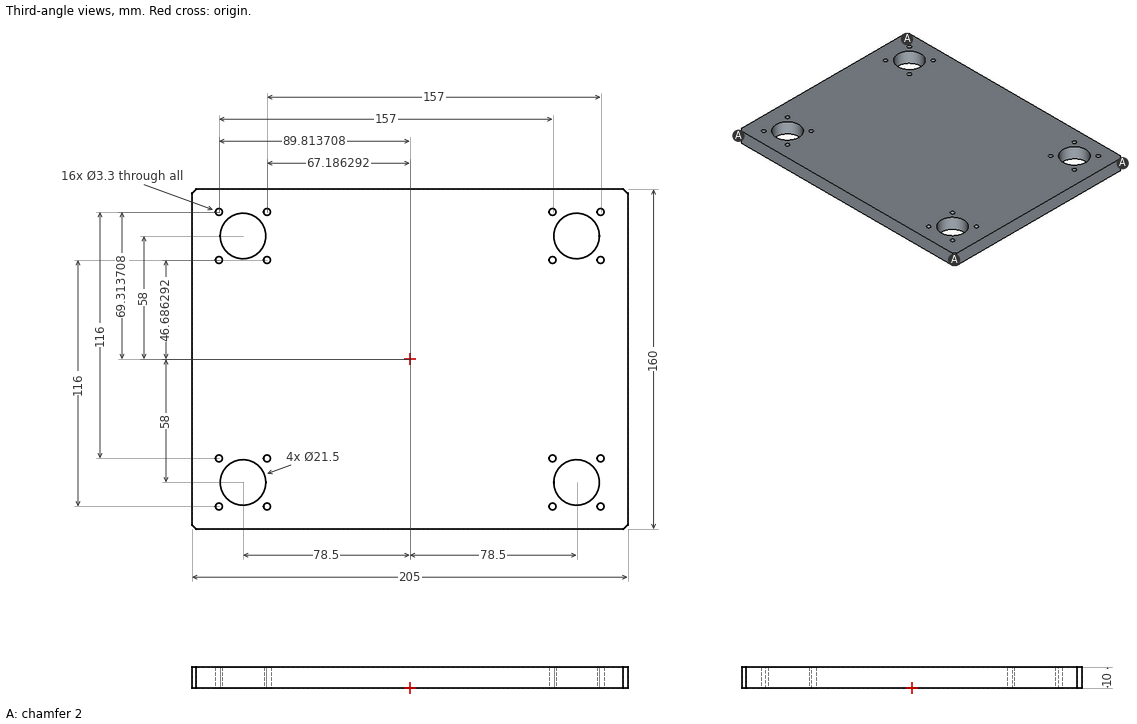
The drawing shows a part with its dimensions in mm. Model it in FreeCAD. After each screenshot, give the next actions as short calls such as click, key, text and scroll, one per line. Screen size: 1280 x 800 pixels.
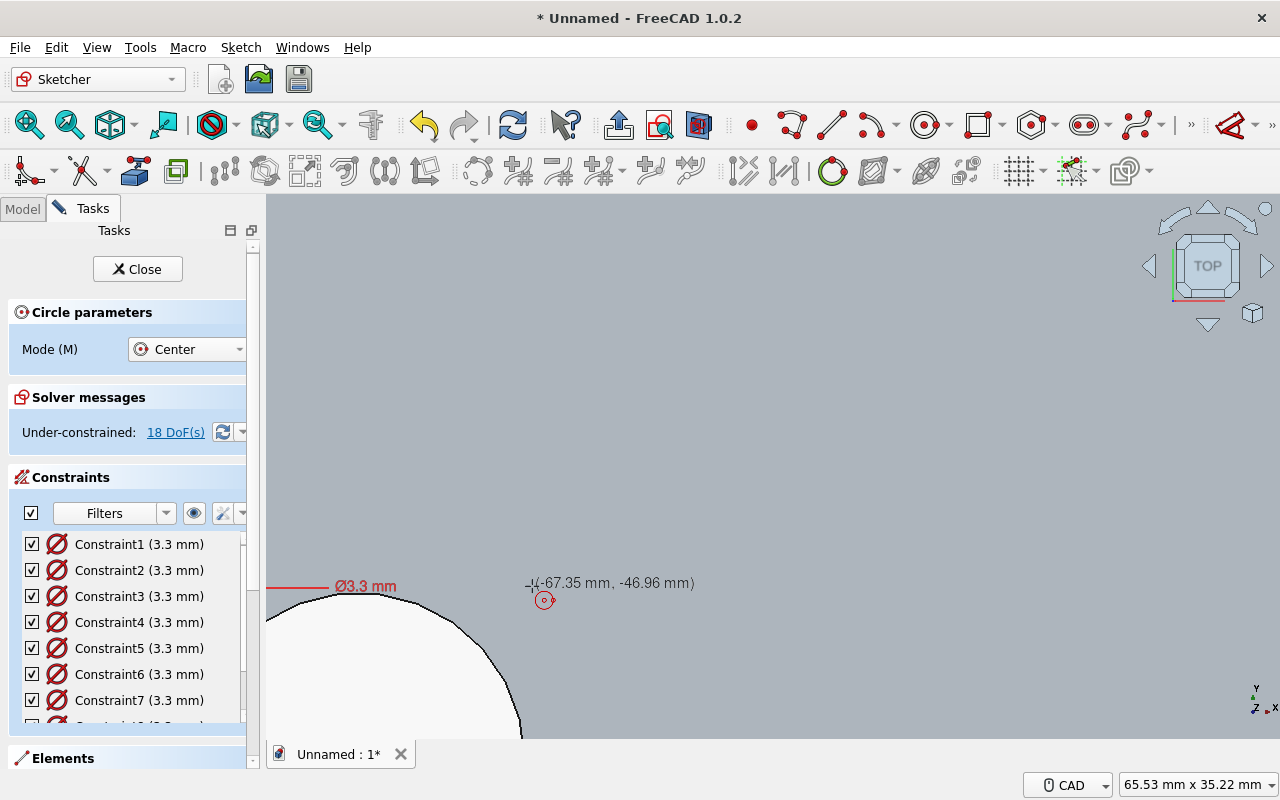
scroll(533, 586, down, 9)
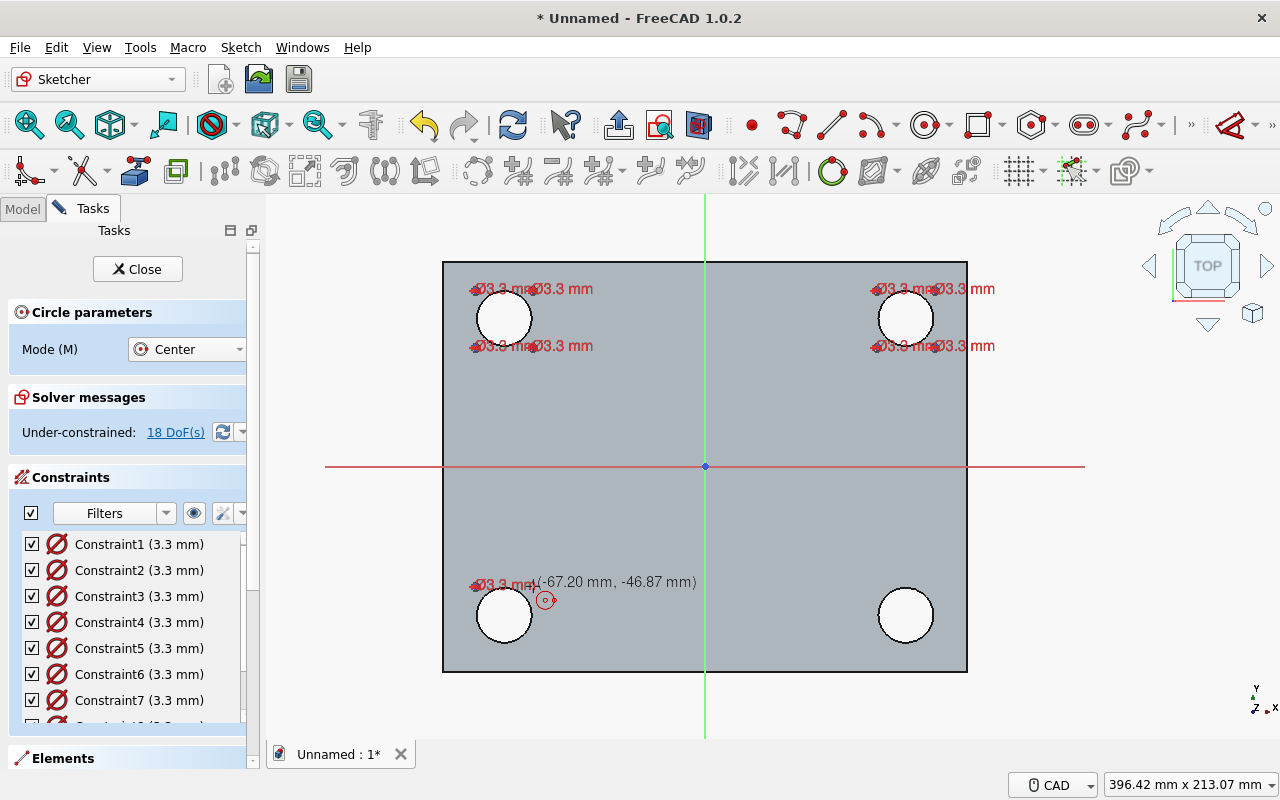
click(533, 586)
move(536, 583)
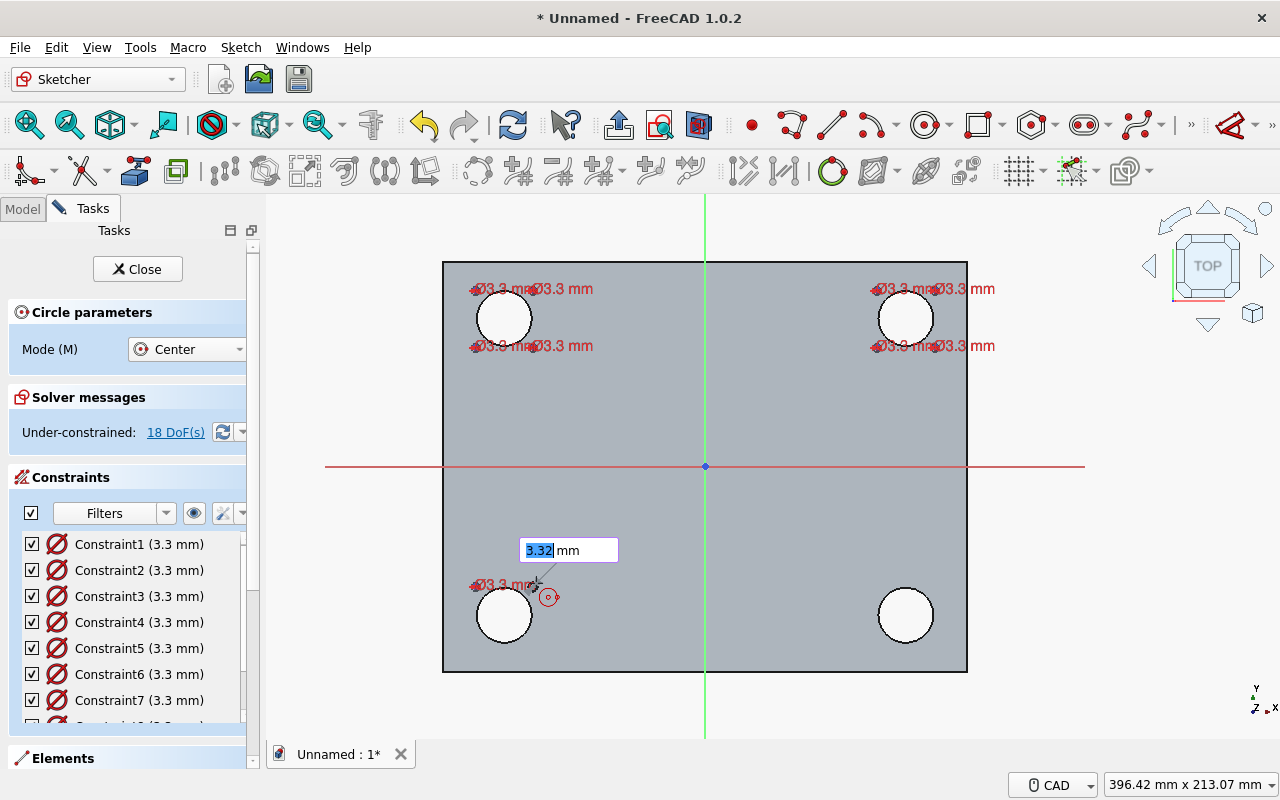
text(3.3)
key(Return)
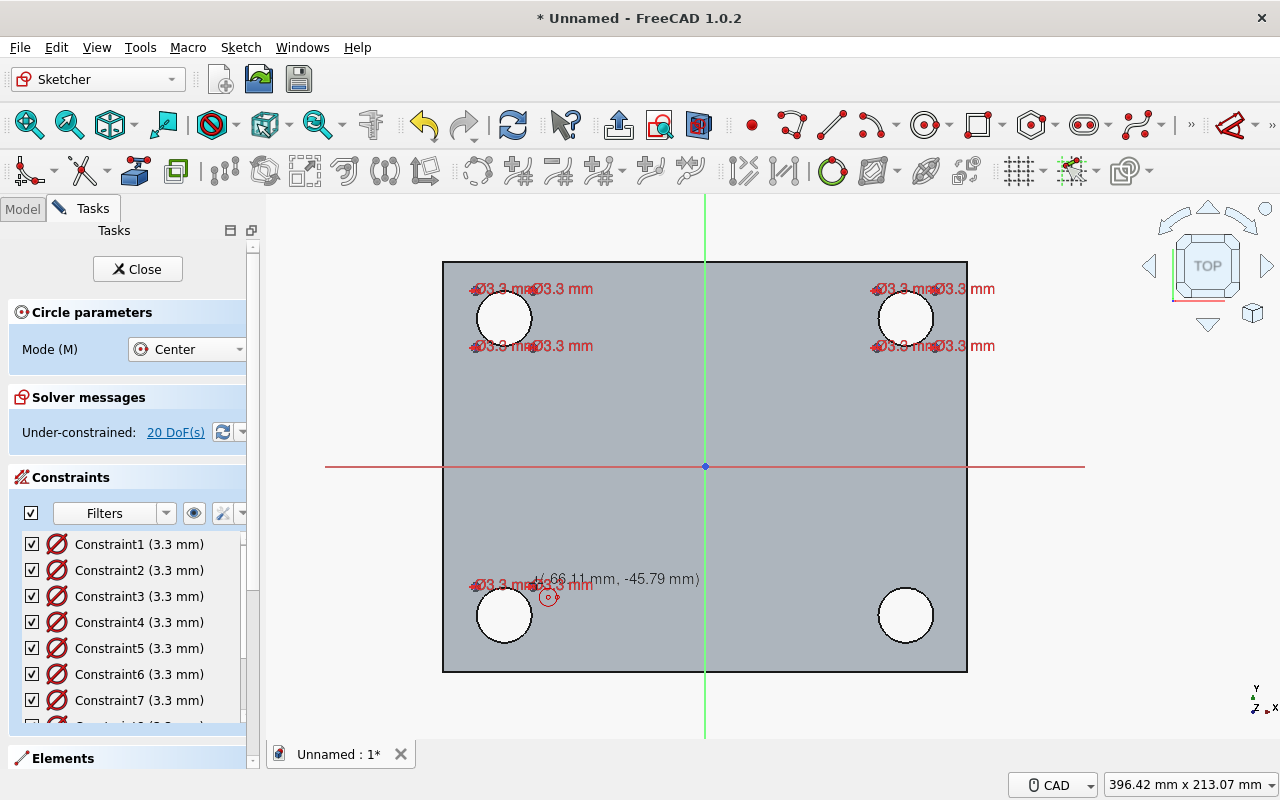
scroll(475, 644, up, 9)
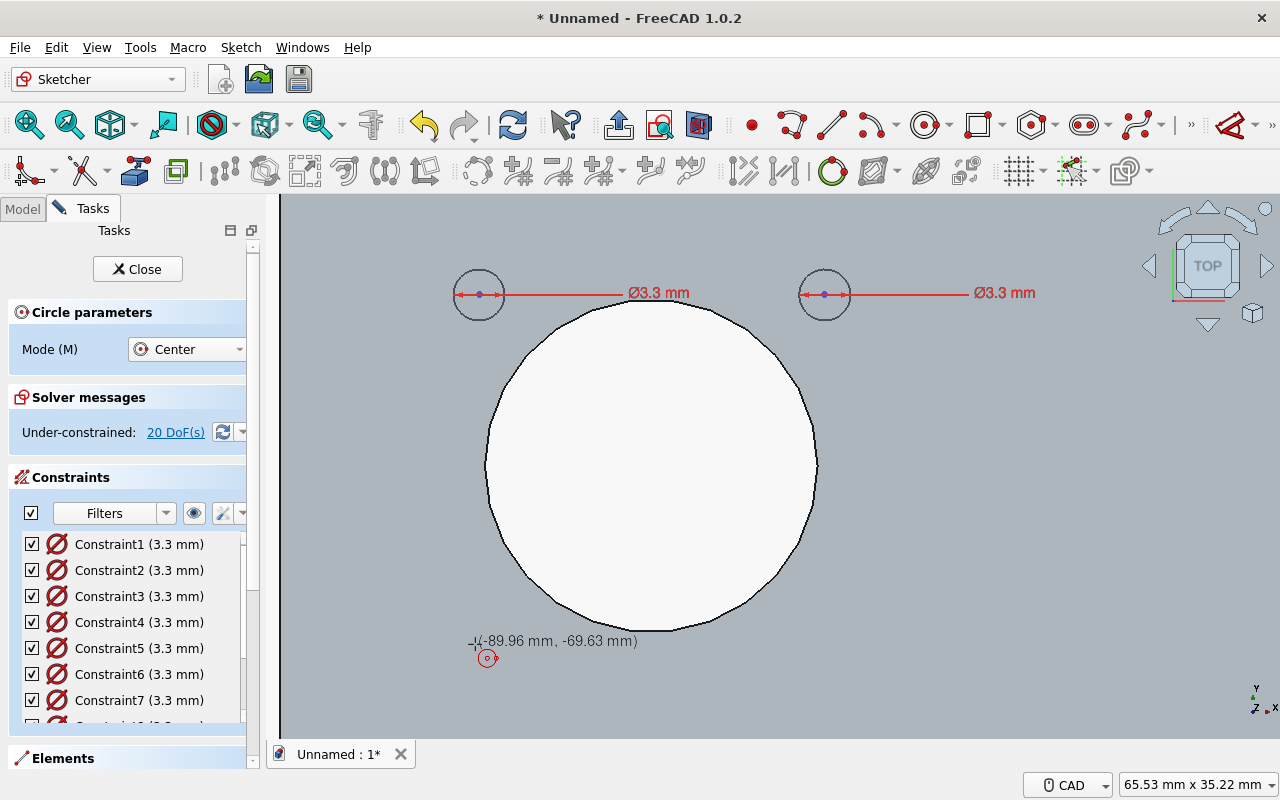
scroll(474, 644, down, 9)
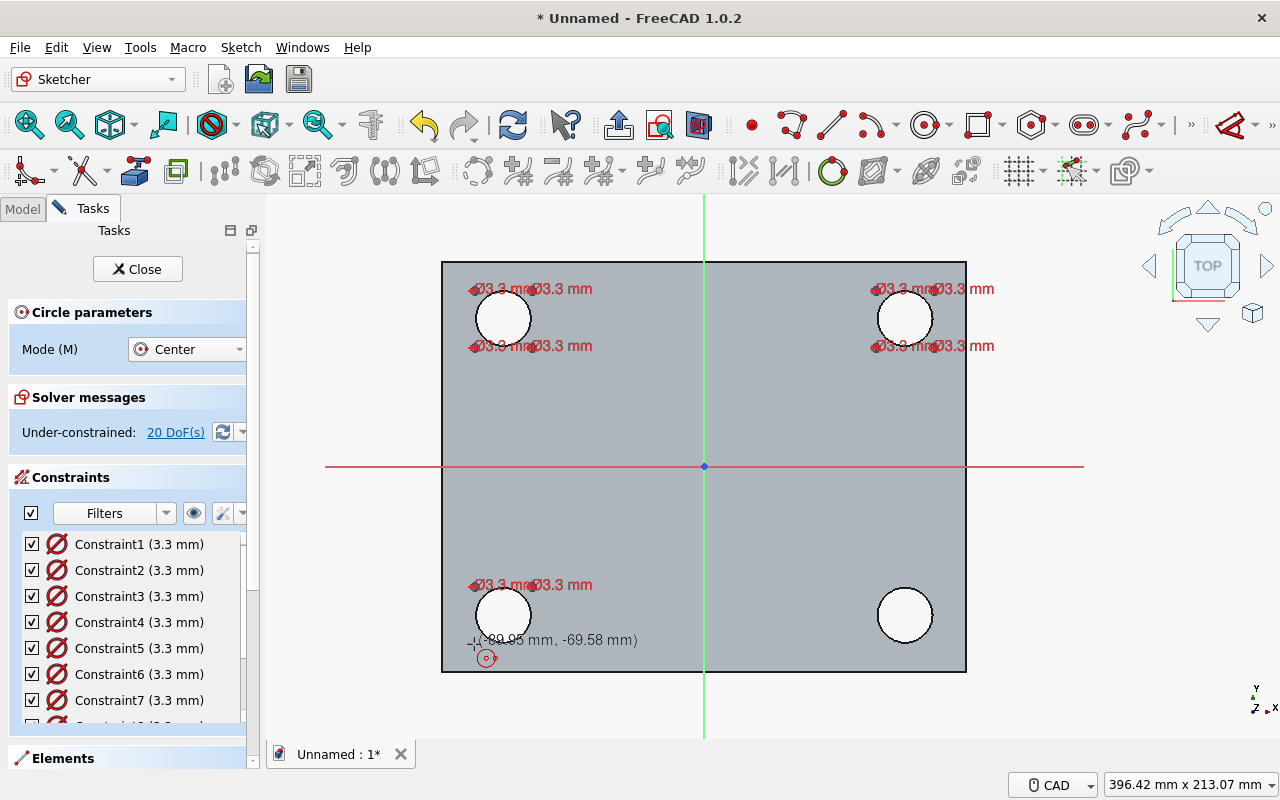
click(475, 644)
move(478, 641)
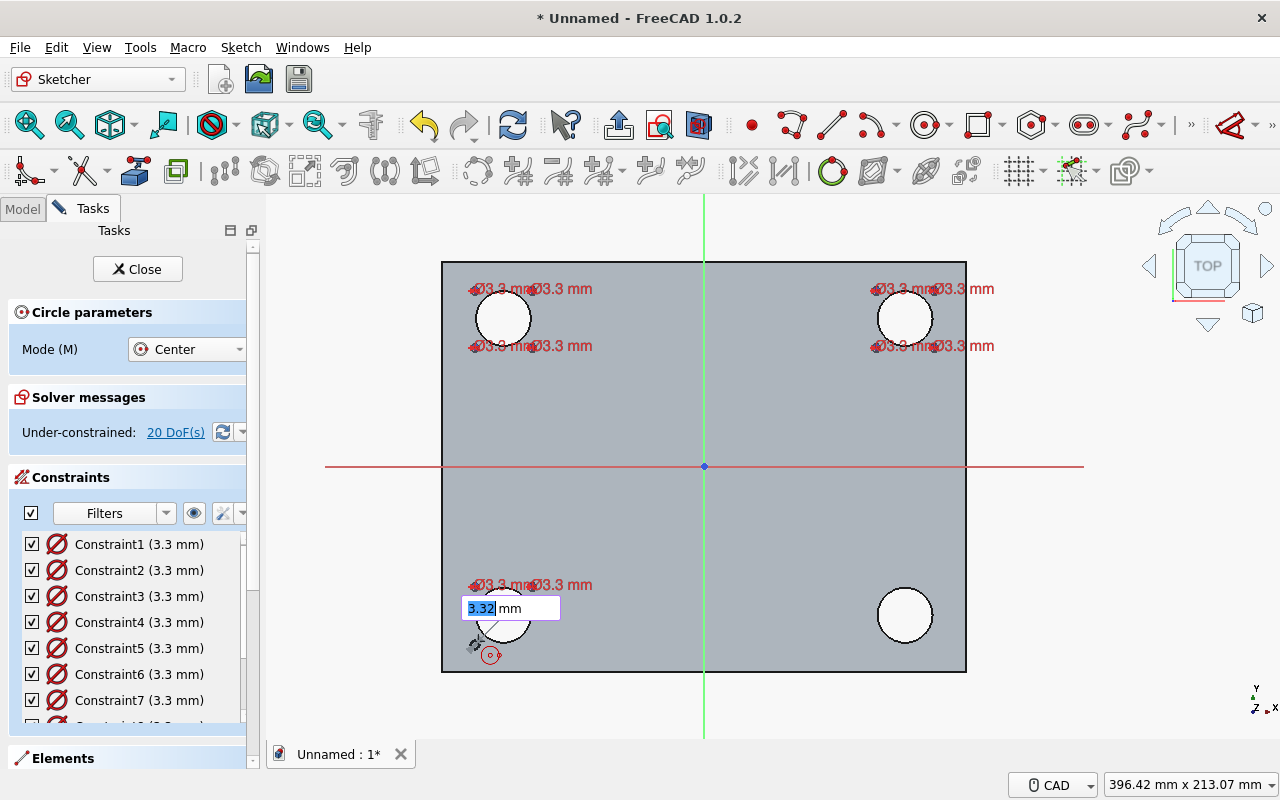
text(3.3)
key(Return)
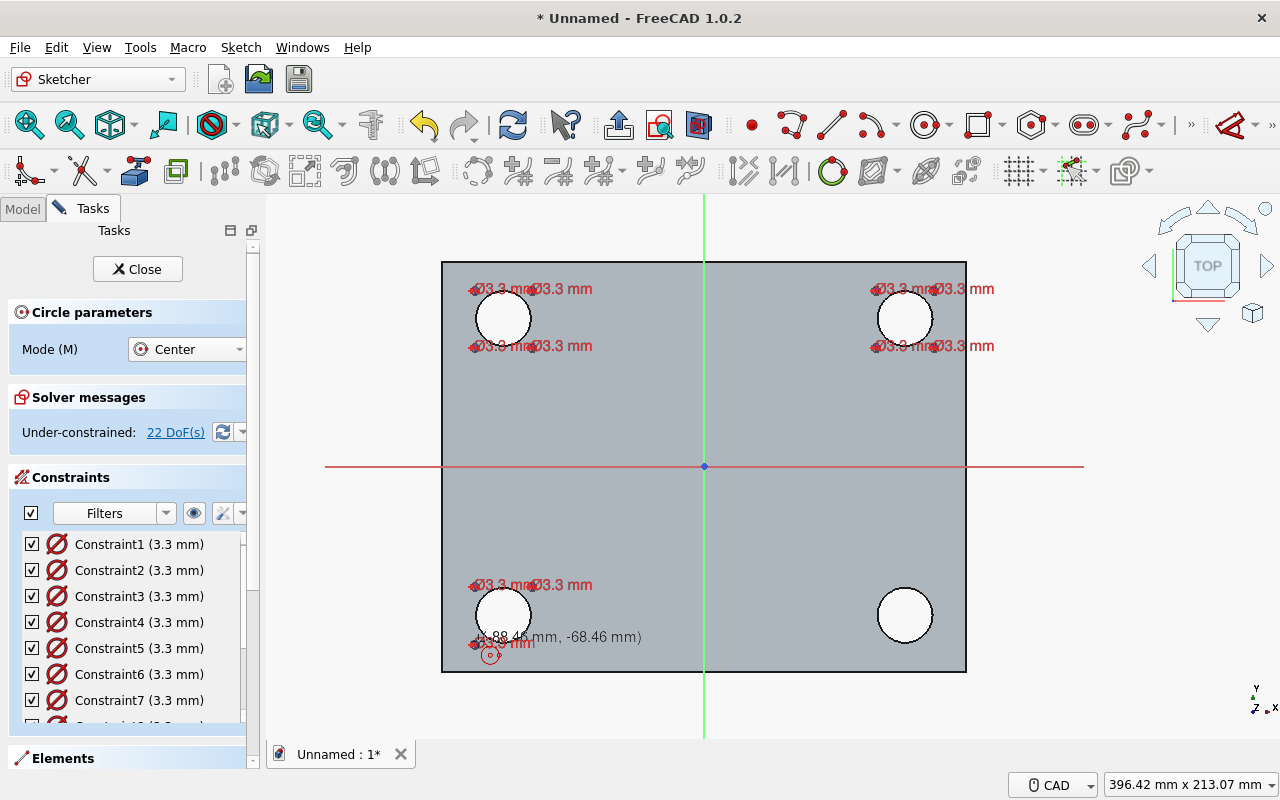
scroll(532, 644, up, 9)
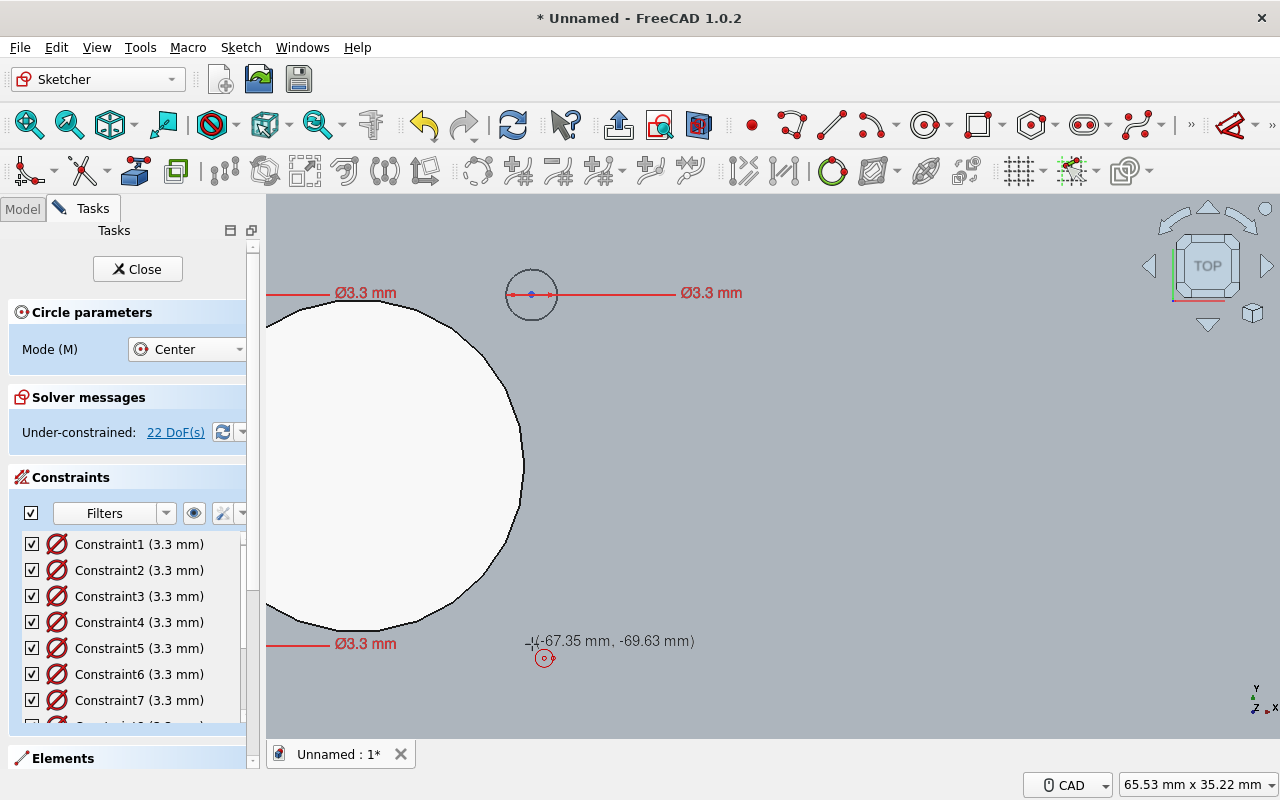
scroll(533, 644, down, 9)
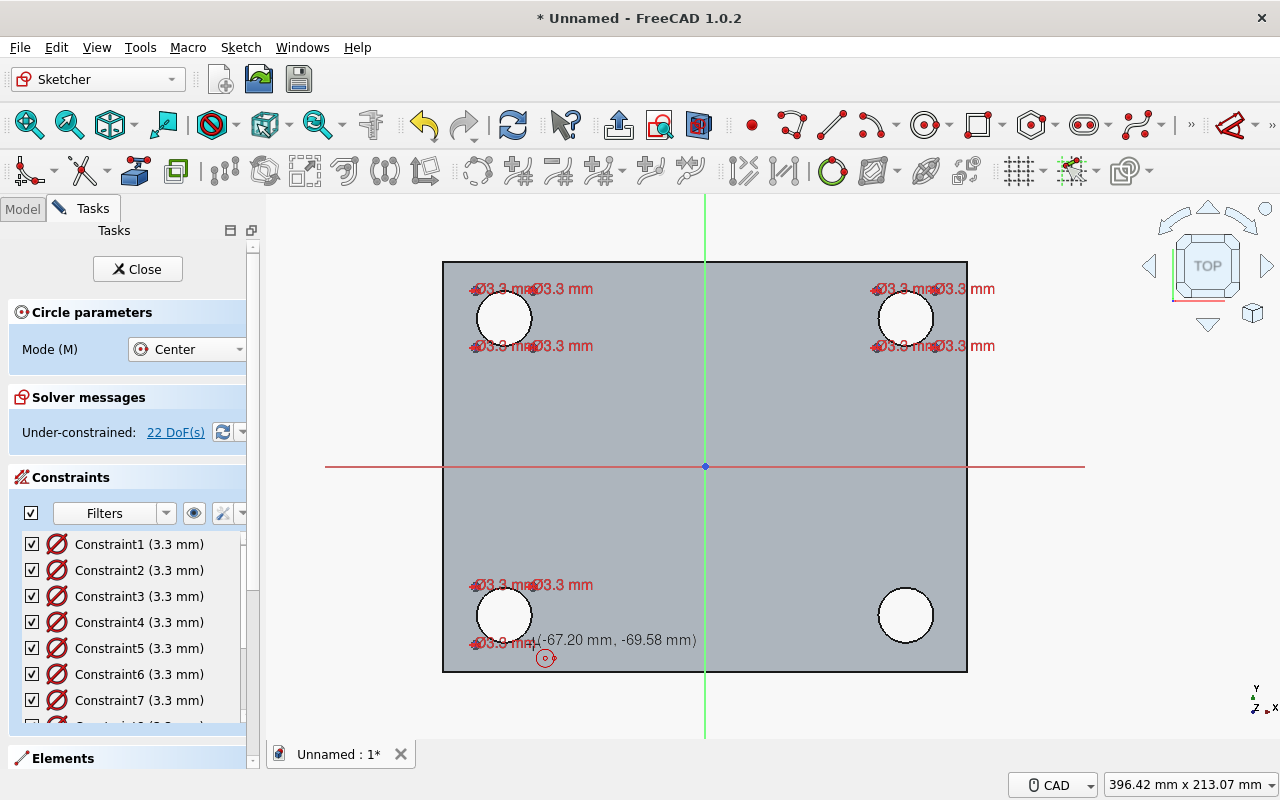
click(533, 644)
move(536, 641)